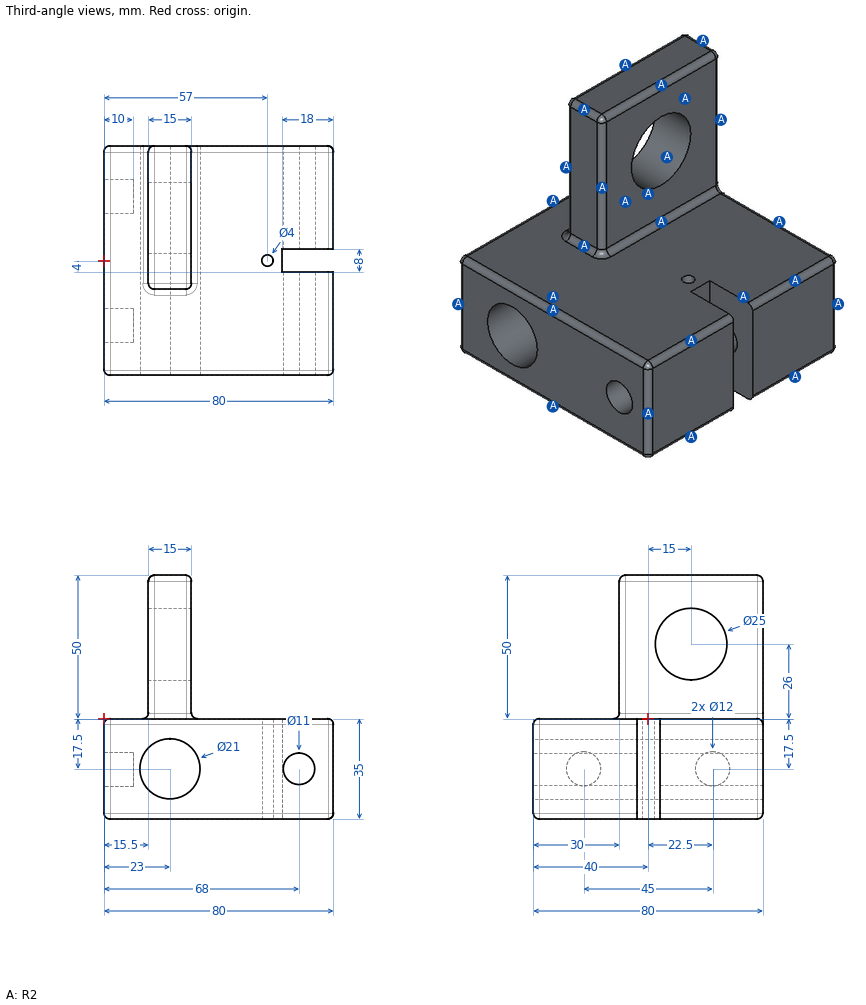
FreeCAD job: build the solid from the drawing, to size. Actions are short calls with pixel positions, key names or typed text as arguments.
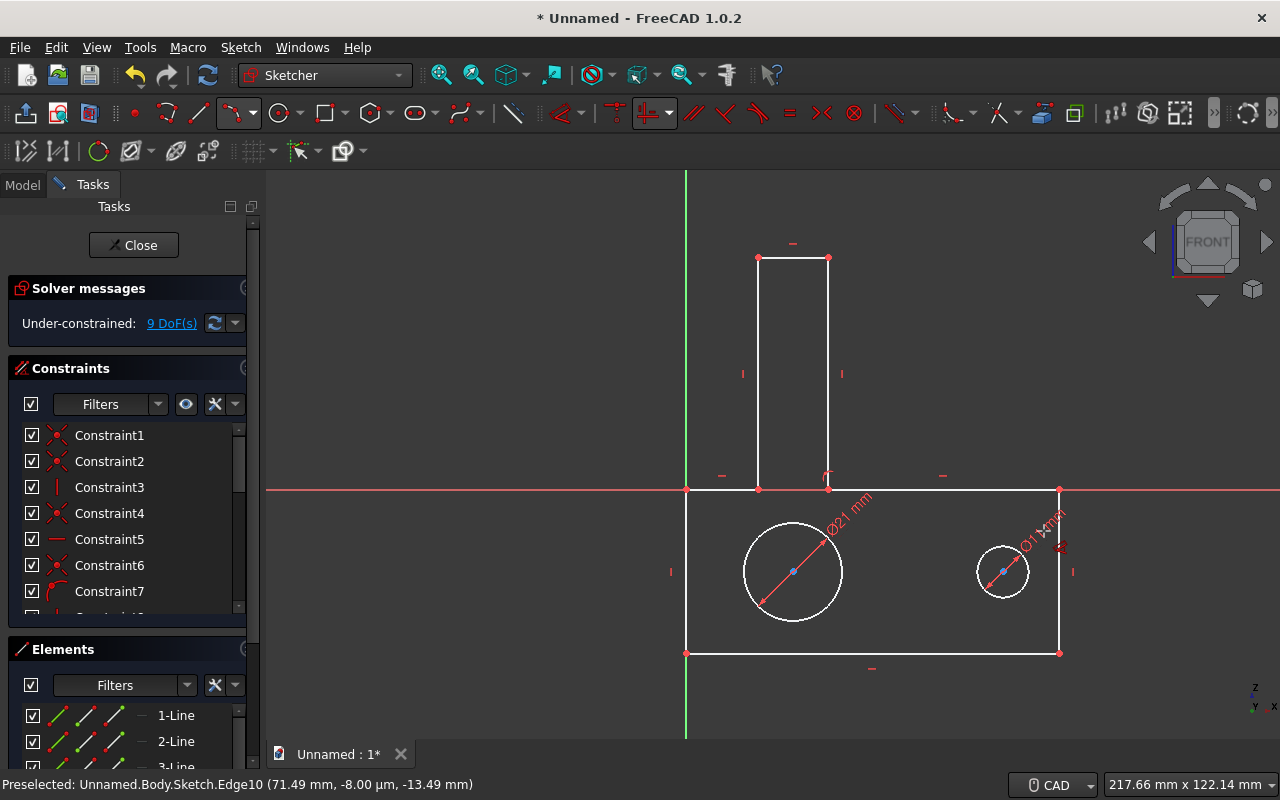
click(758, 420)
click(724, 374)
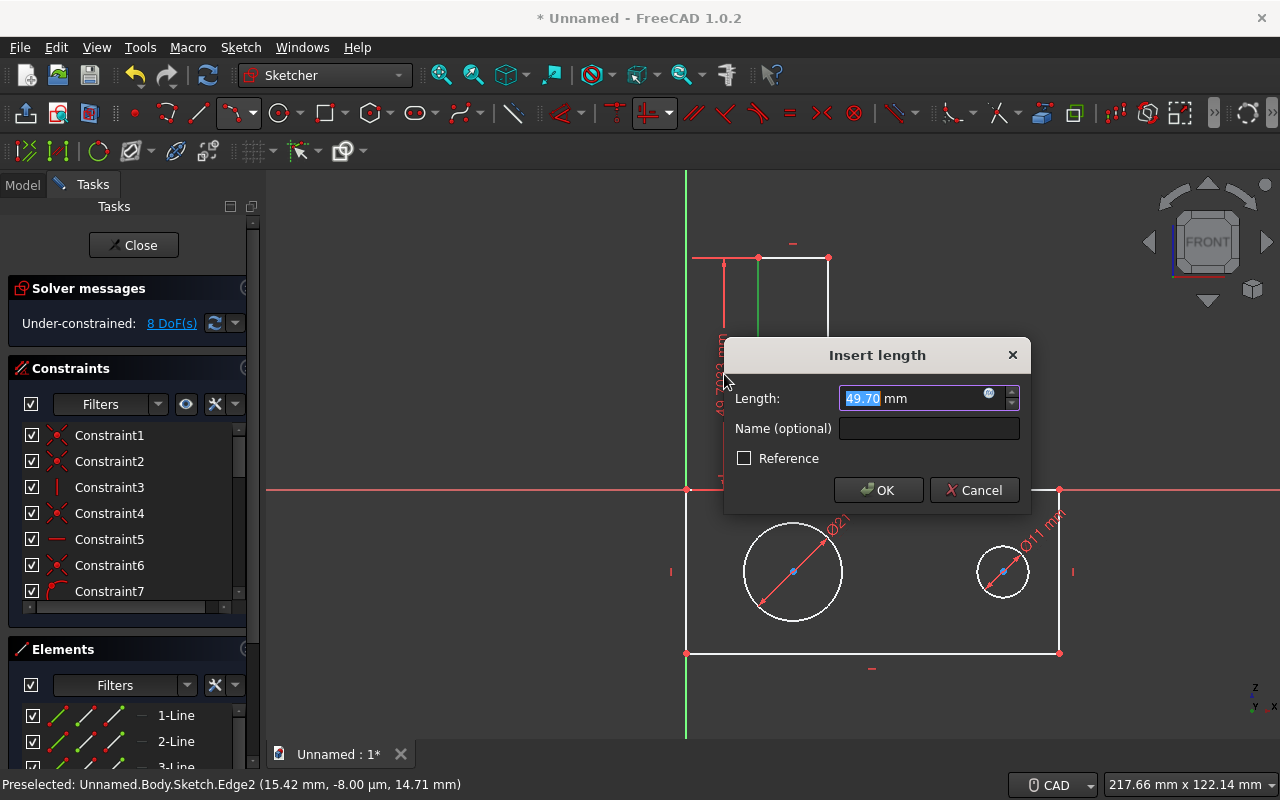
text(50)
key(Return)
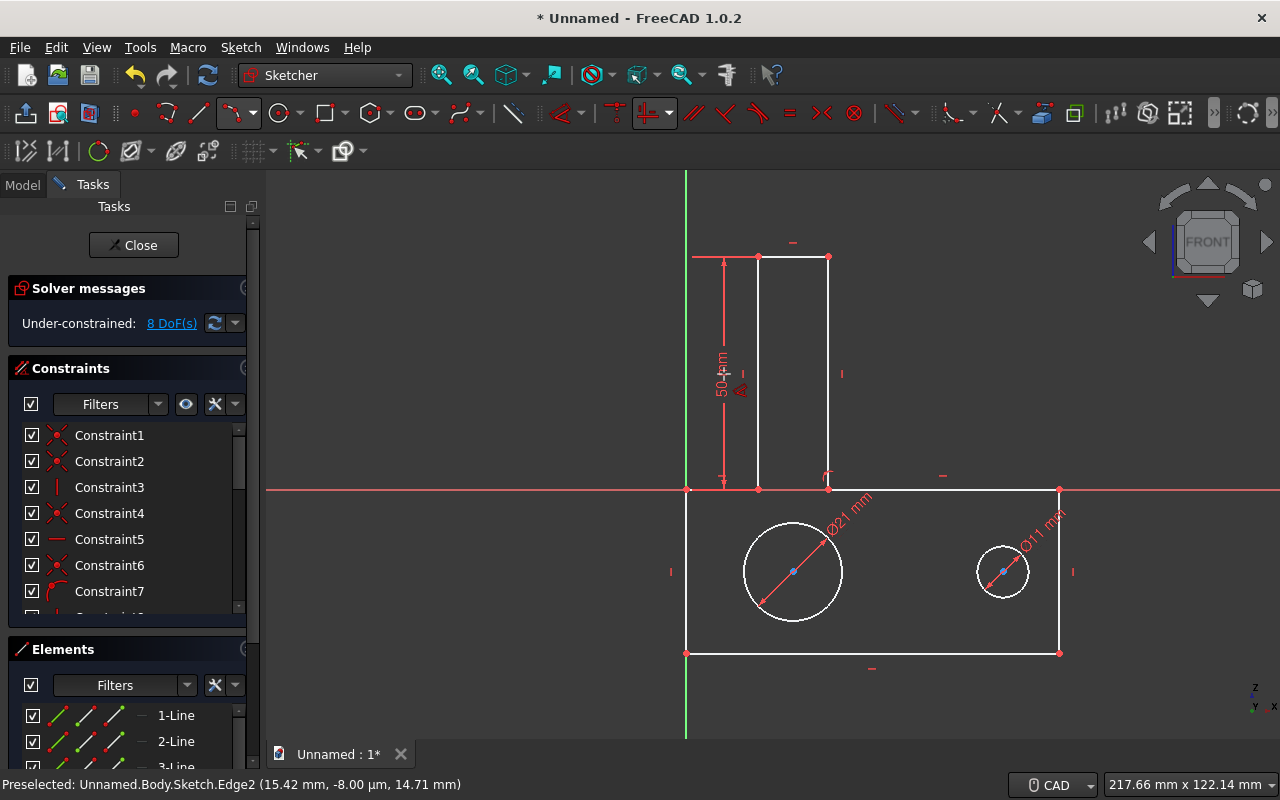
click(779, 257)
click(793, 223)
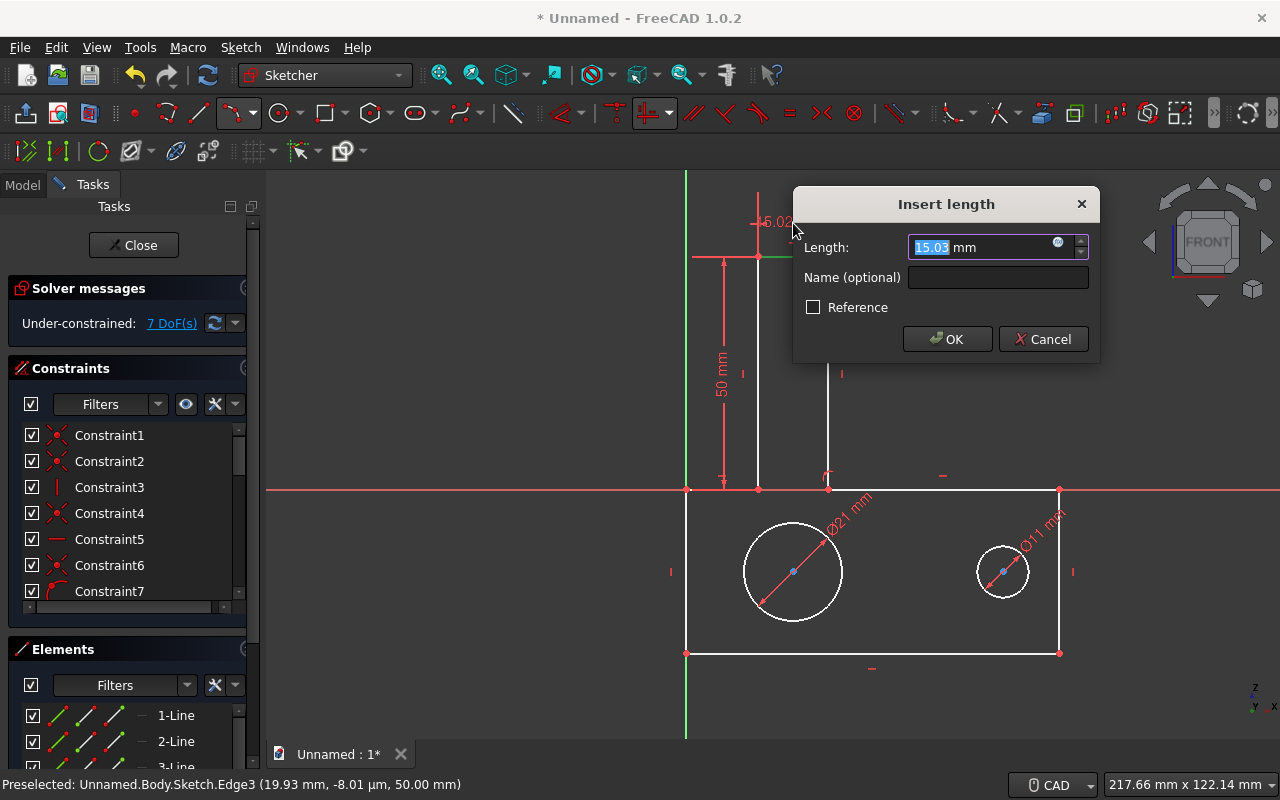
text(15)
key(Return)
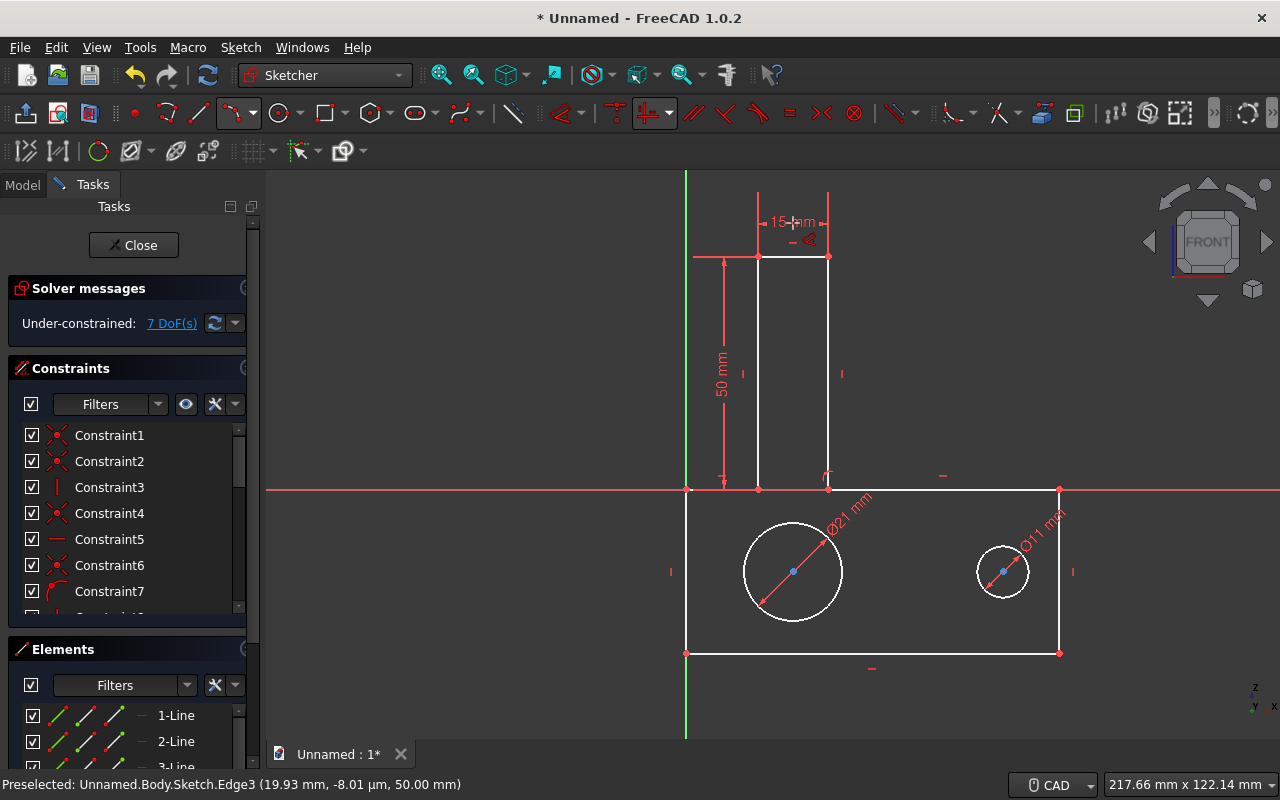
click(1059, 539)
click(1093, 572)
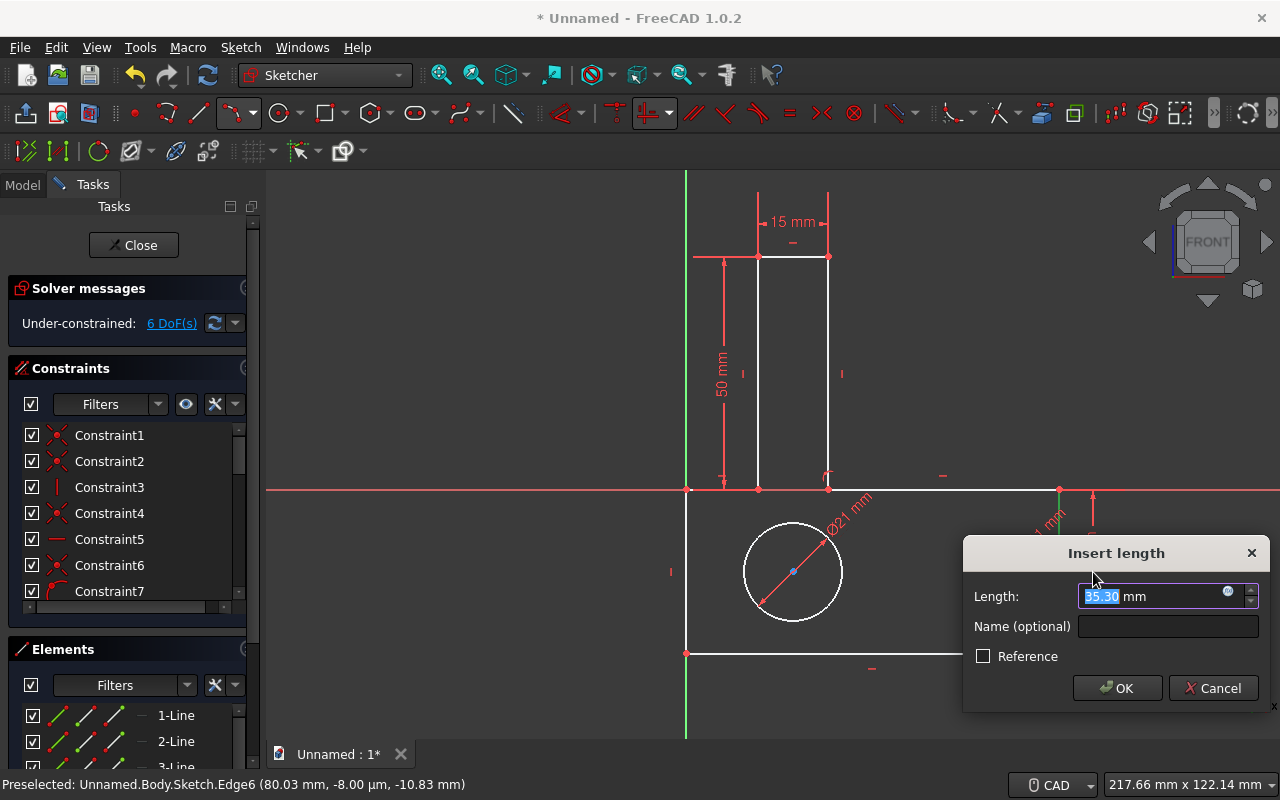
text(35)
key(Return)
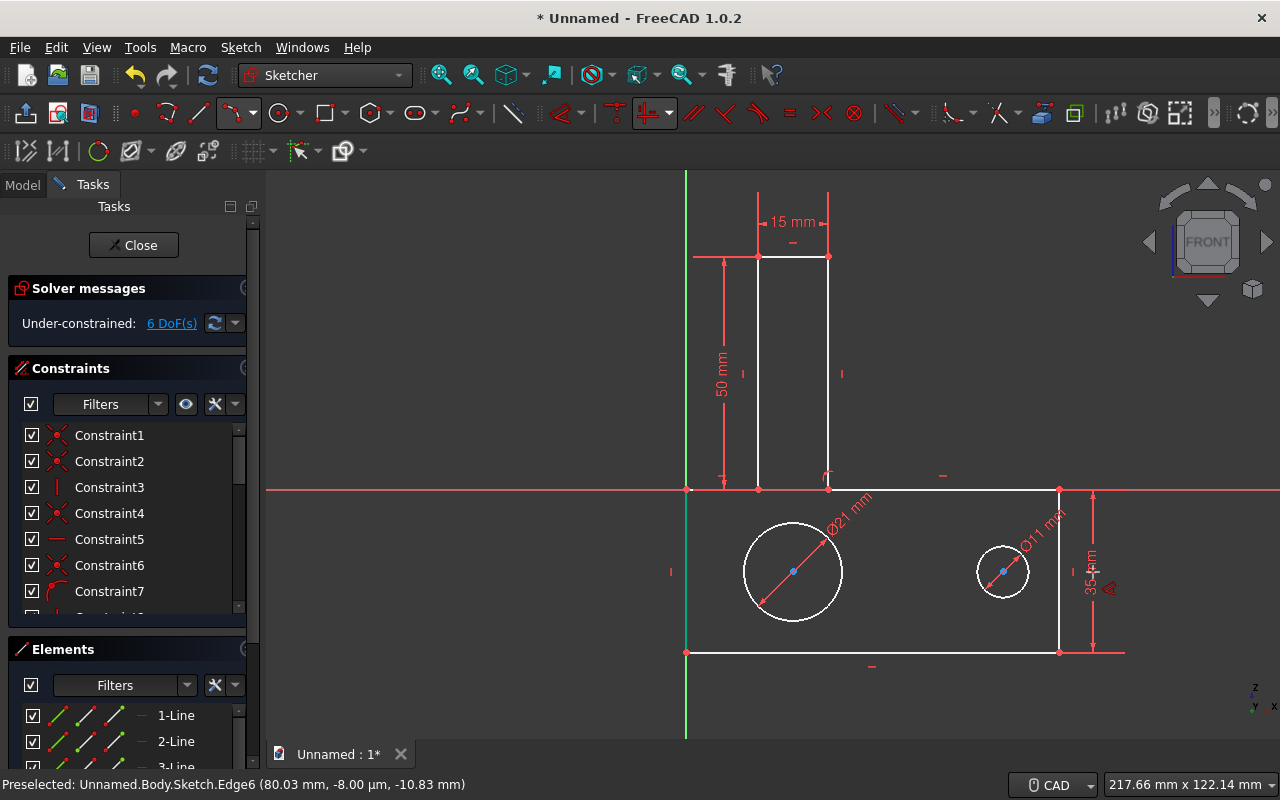
click(947, 653)
click(873, 687)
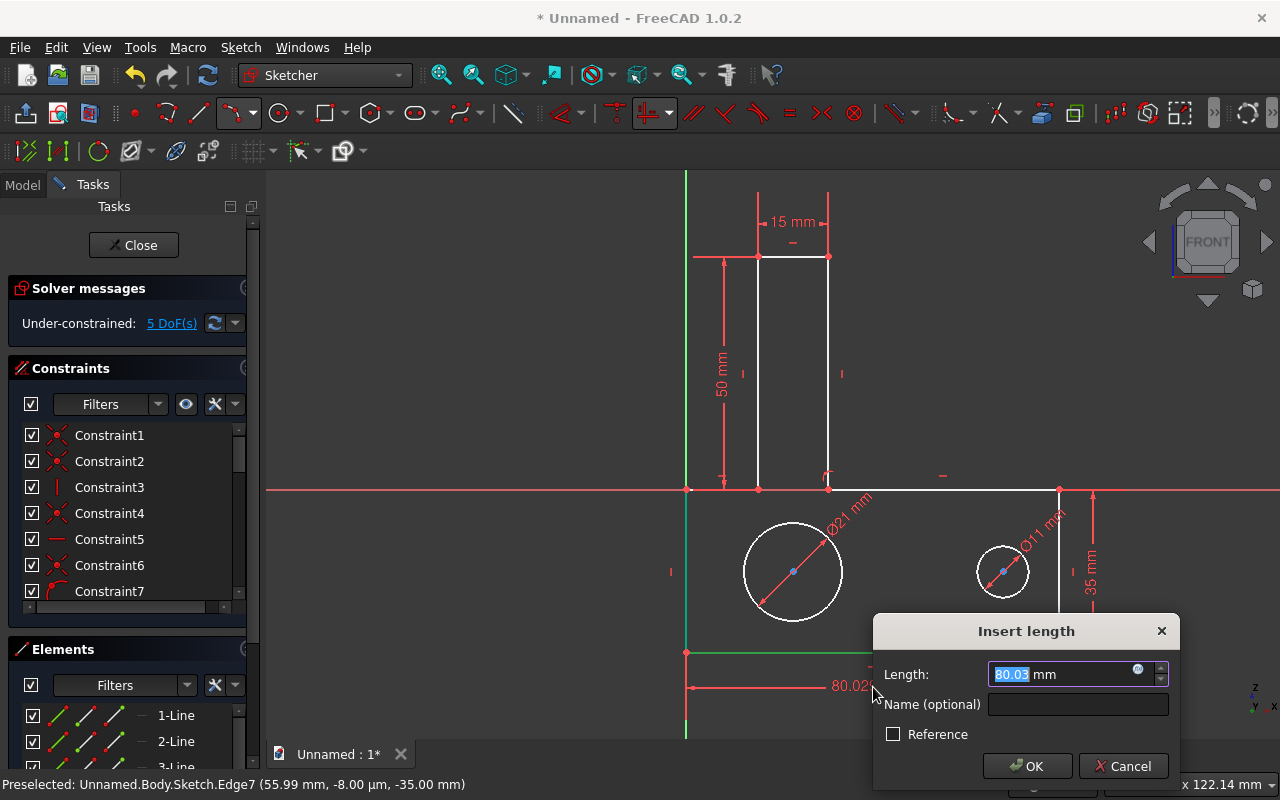
text(80)
key(Return)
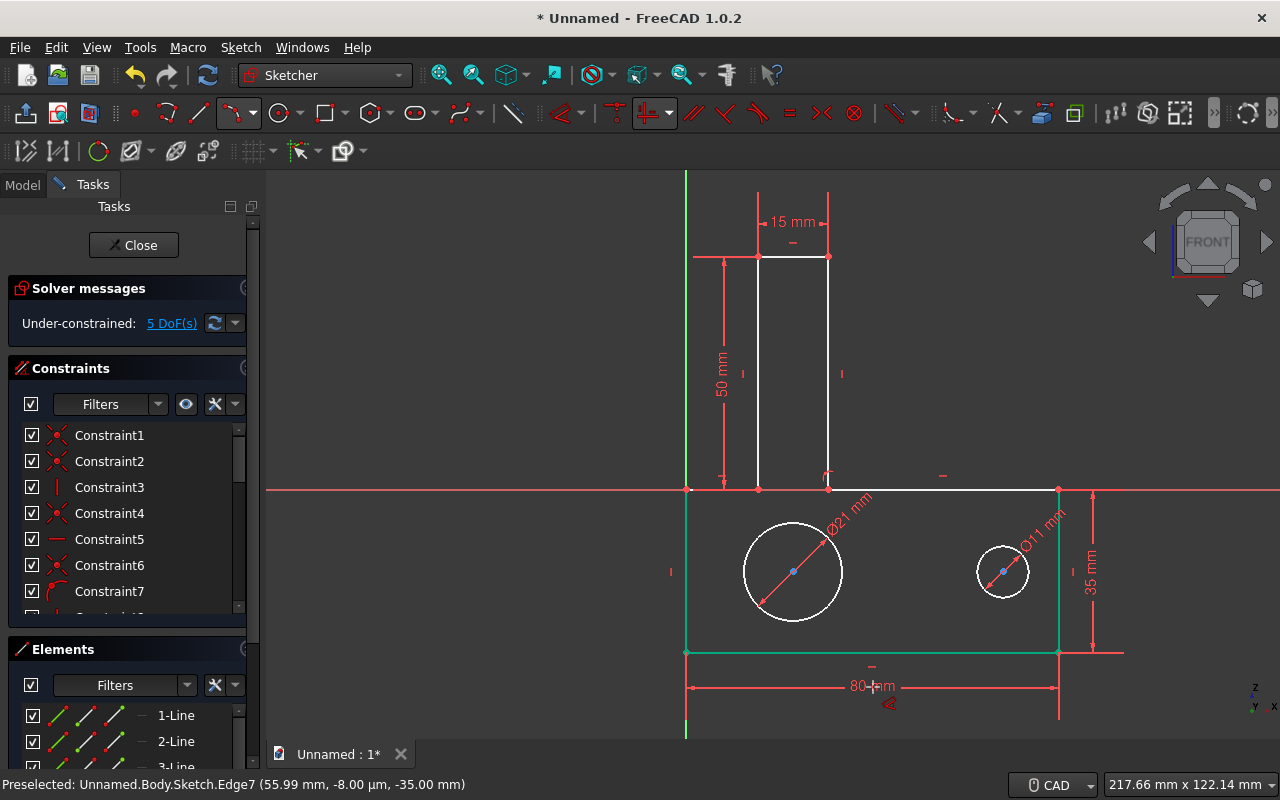
click(793, 572)
click(740, 606)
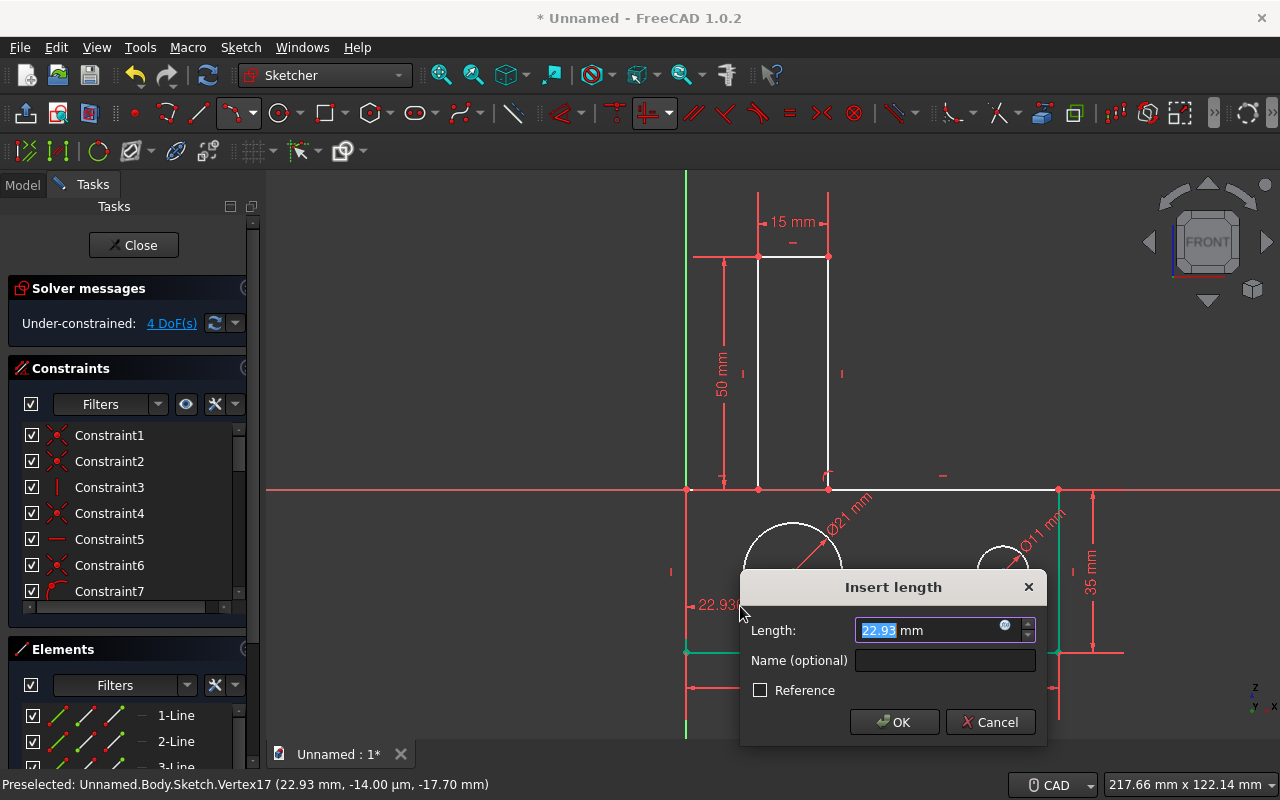
text(23)
key(Return)